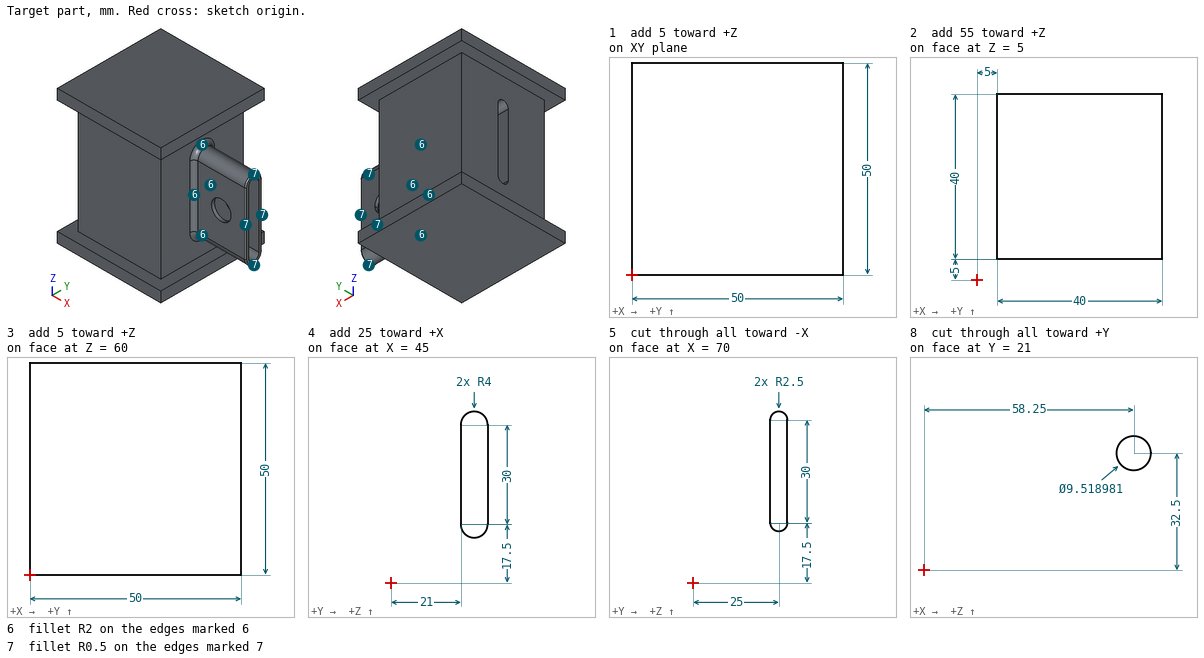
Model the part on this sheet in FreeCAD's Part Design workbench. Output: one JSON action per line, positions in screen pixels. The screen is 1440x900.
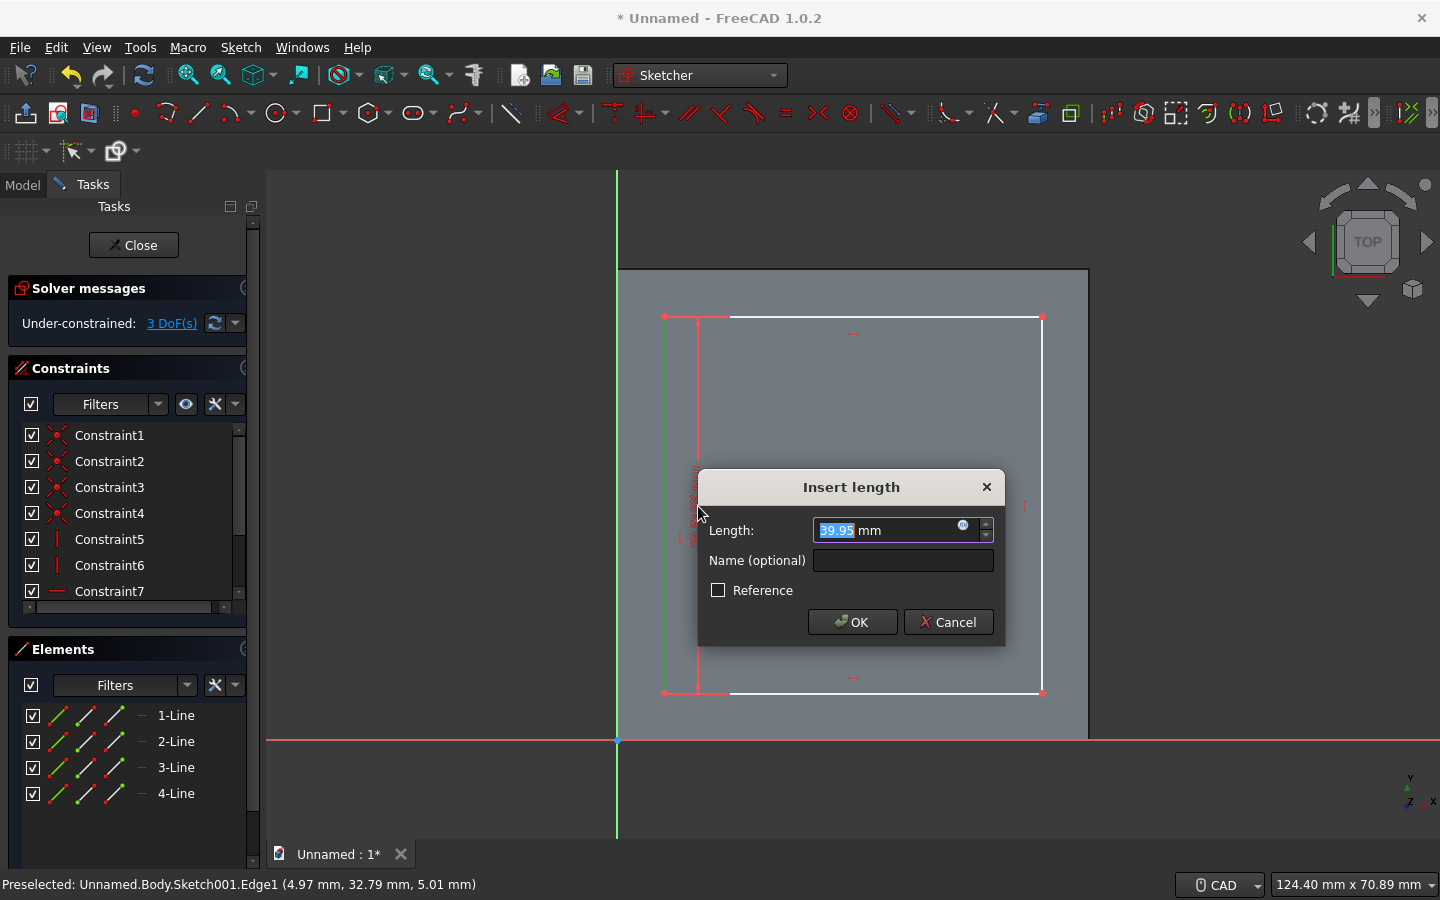
{"action": "type", "text": "40"}
{"action": "key", "text": "Return"}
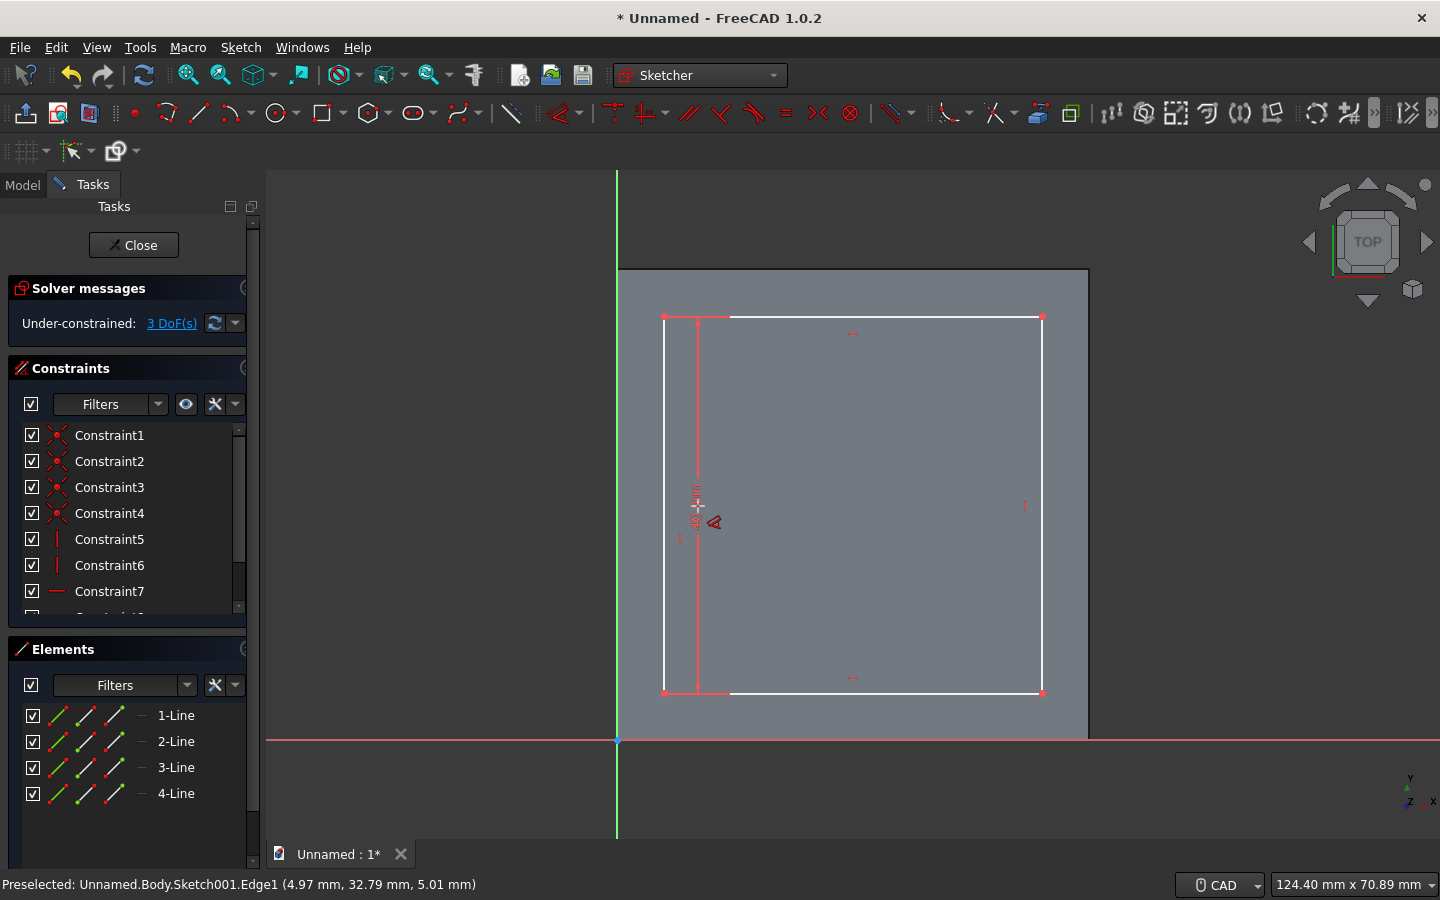
{"action": "left_click", "coordinate": [777, 694]}
{"action": "left_click", "coordinate": [853, 660]}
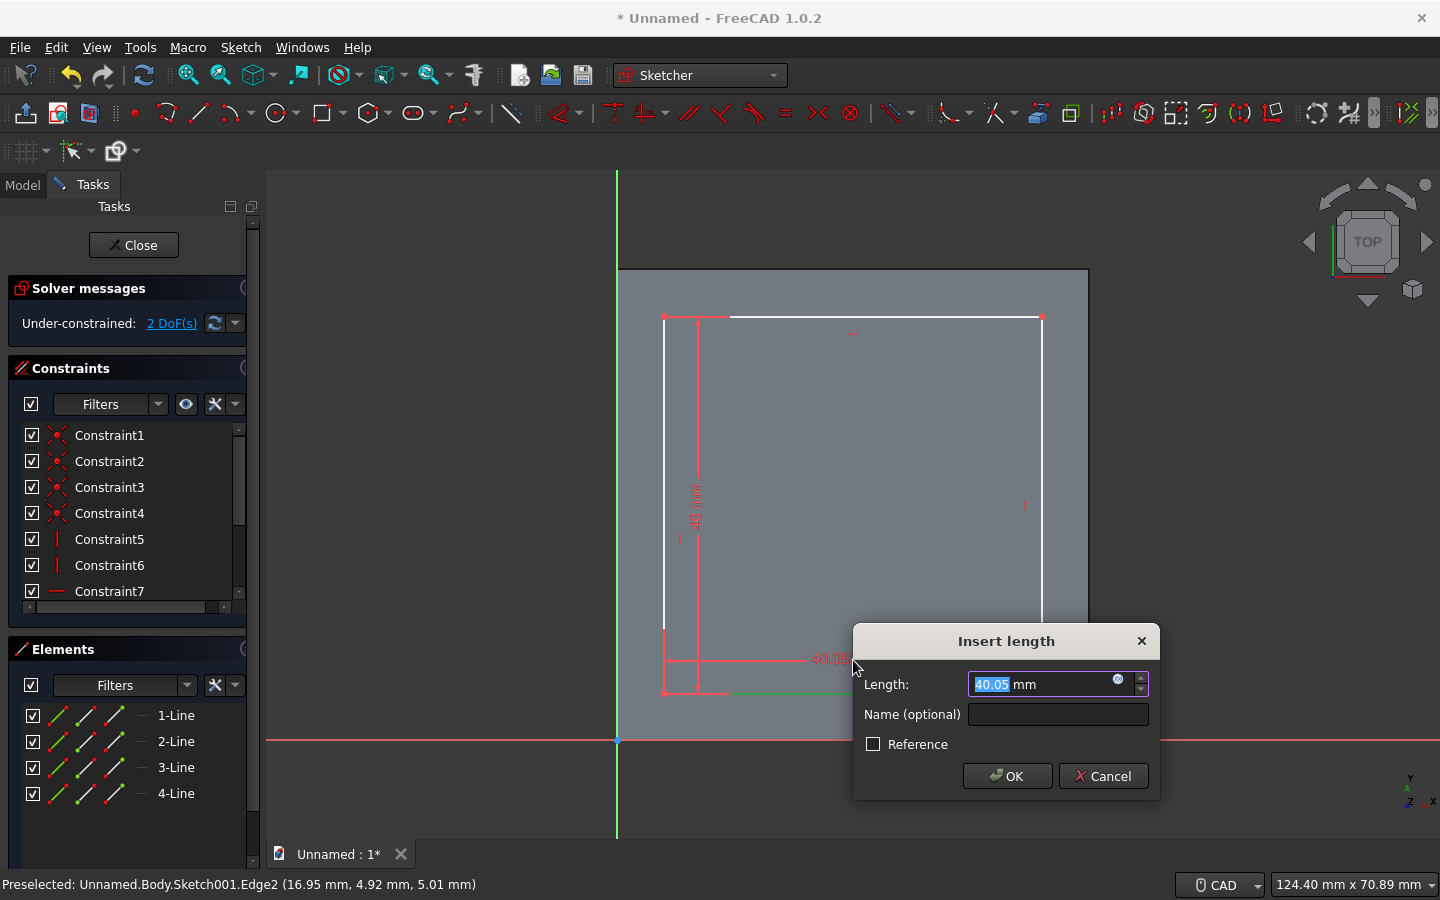
{"action": "type", "text": "40"}
{"action": "key", "text": "Return"}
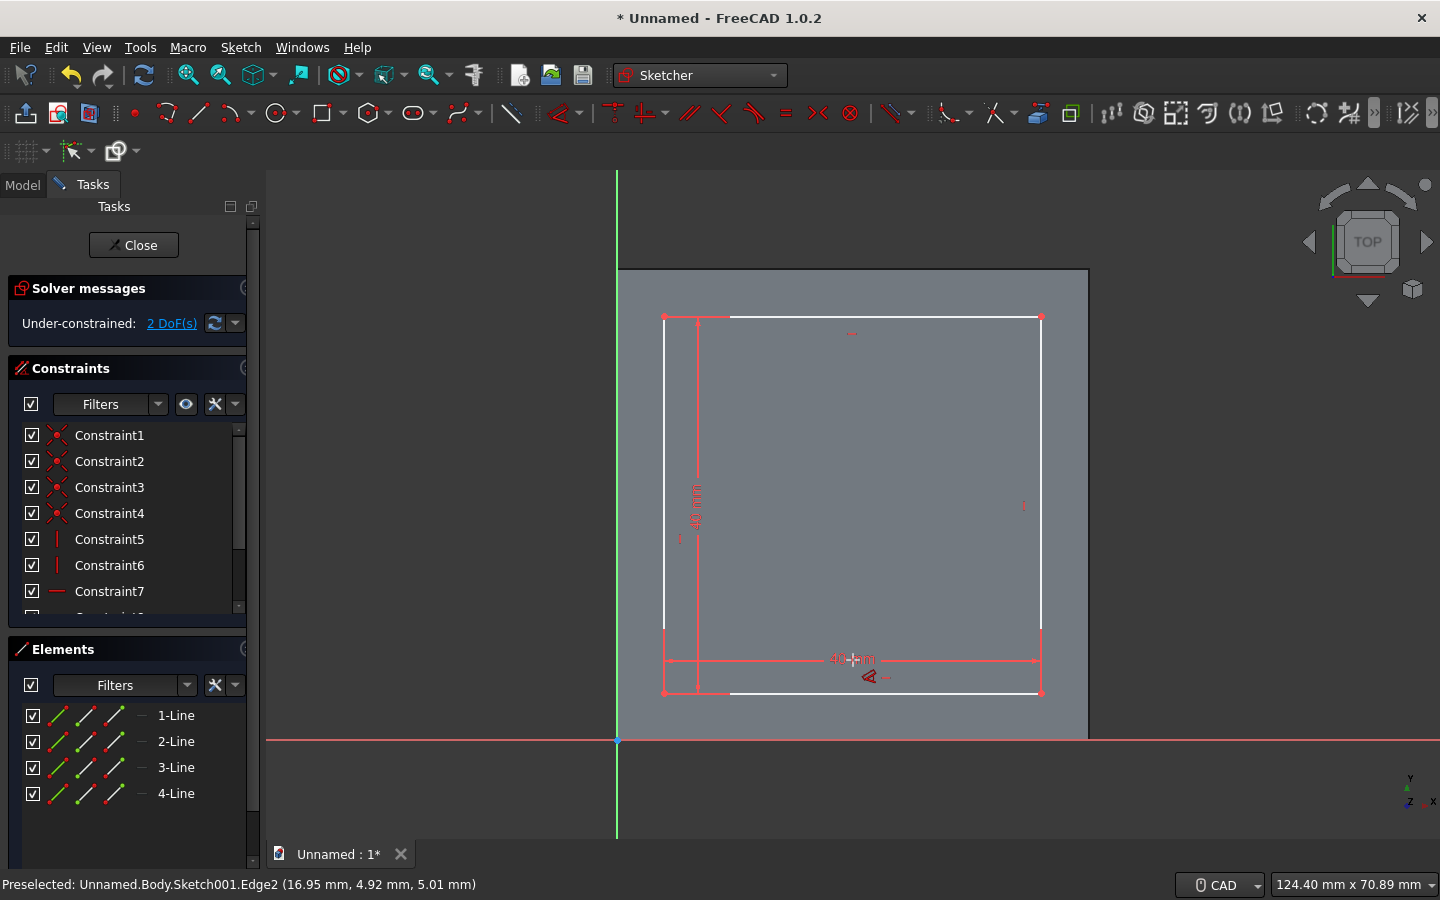
{"action": "left_click", "coordinate": [664, 316]}
{"action": "left_click", "coordinate": [641, 774]}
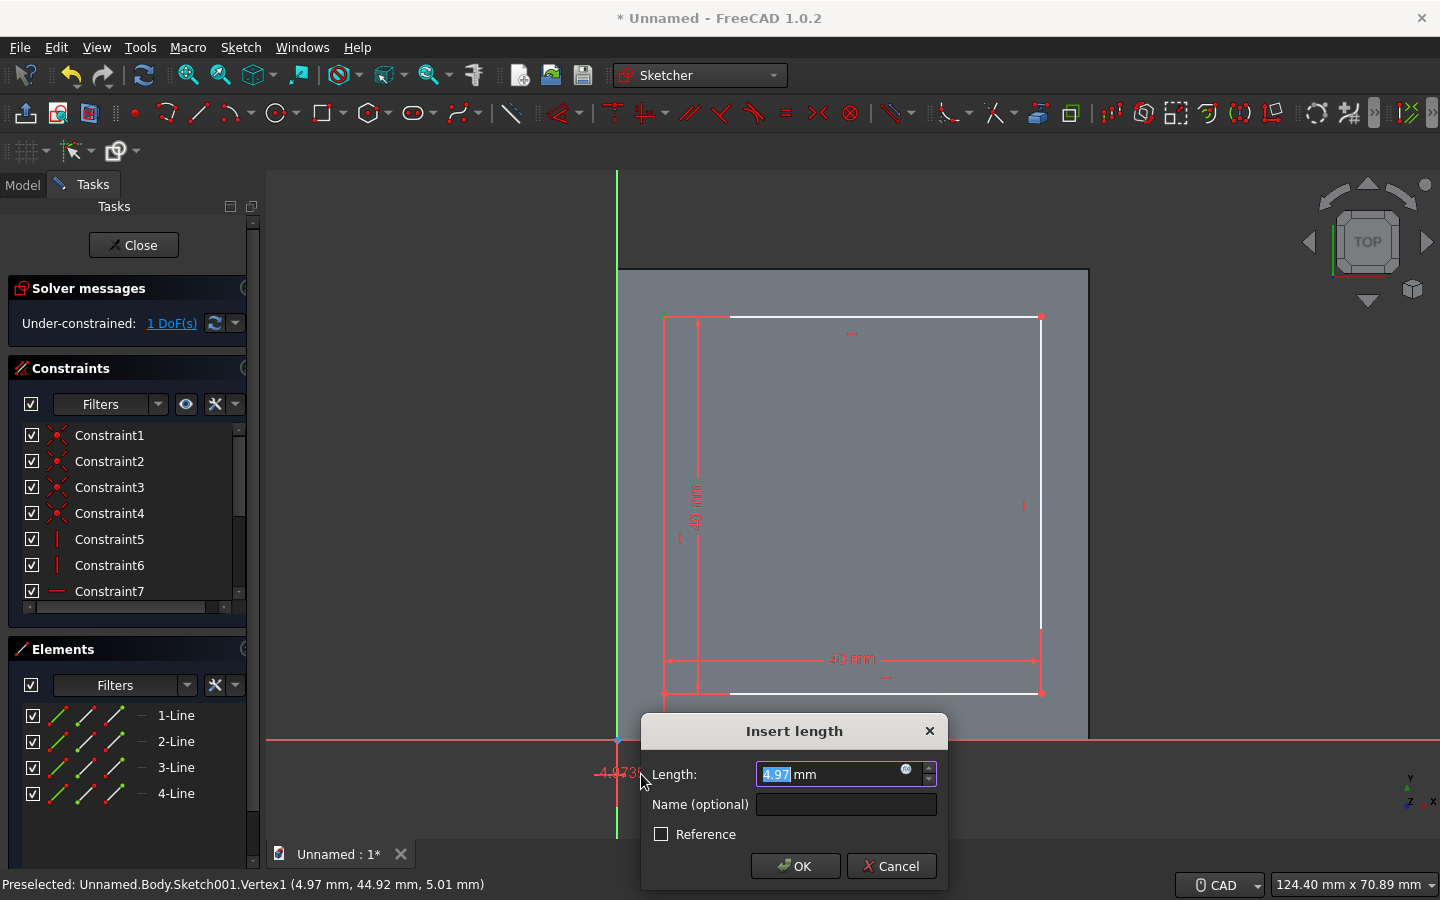
{"action": "type", "text": "5"}
{"action": "key", "text": "Return"}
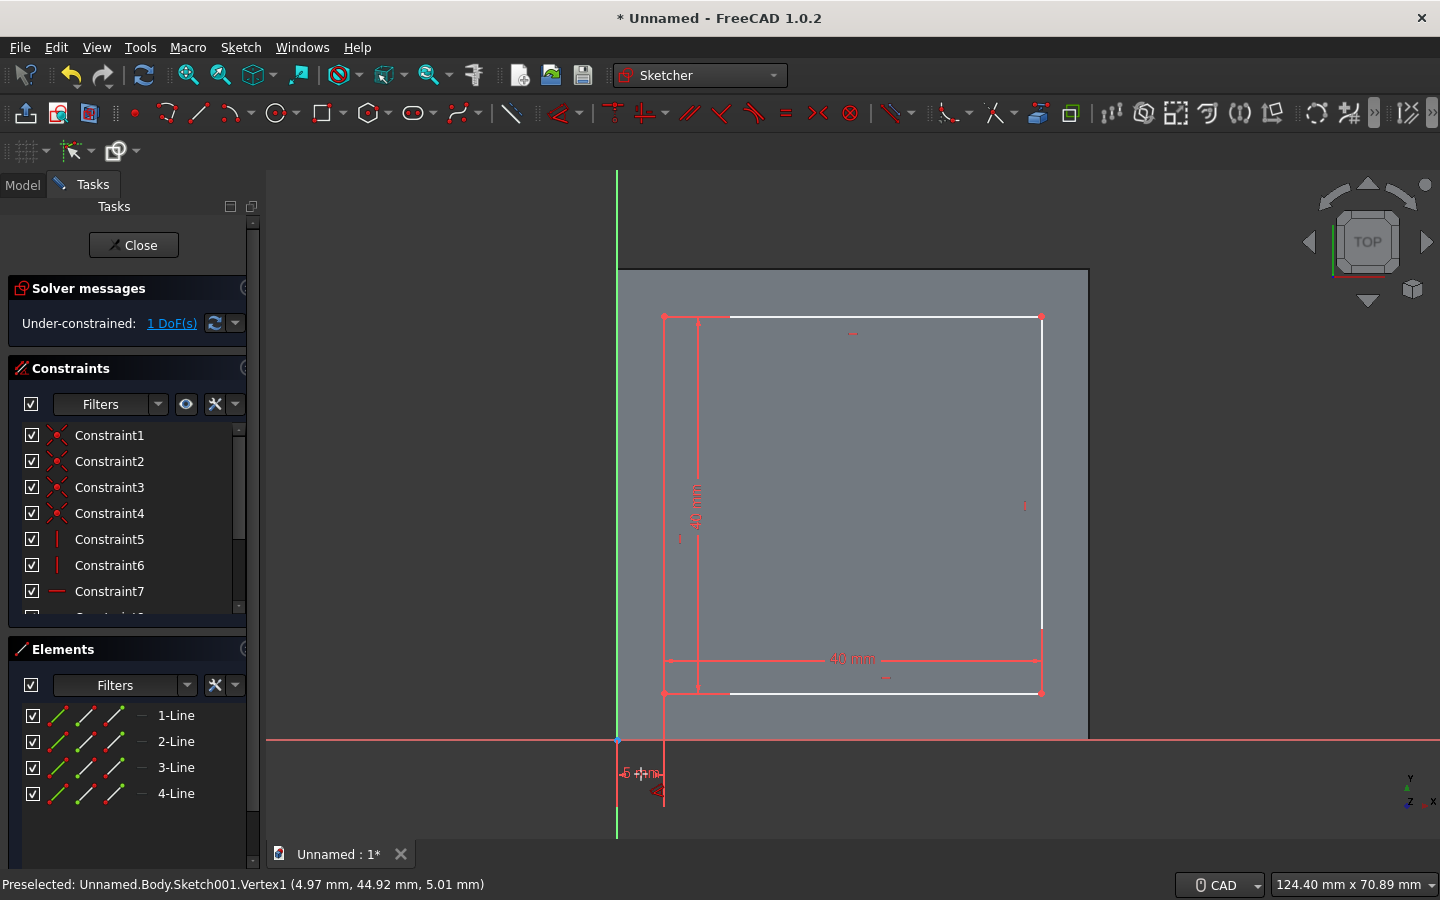
{"action": "left_click", "coordinate": [664, 694]}
{"action": "left_click", "coordinate": [583, 717]}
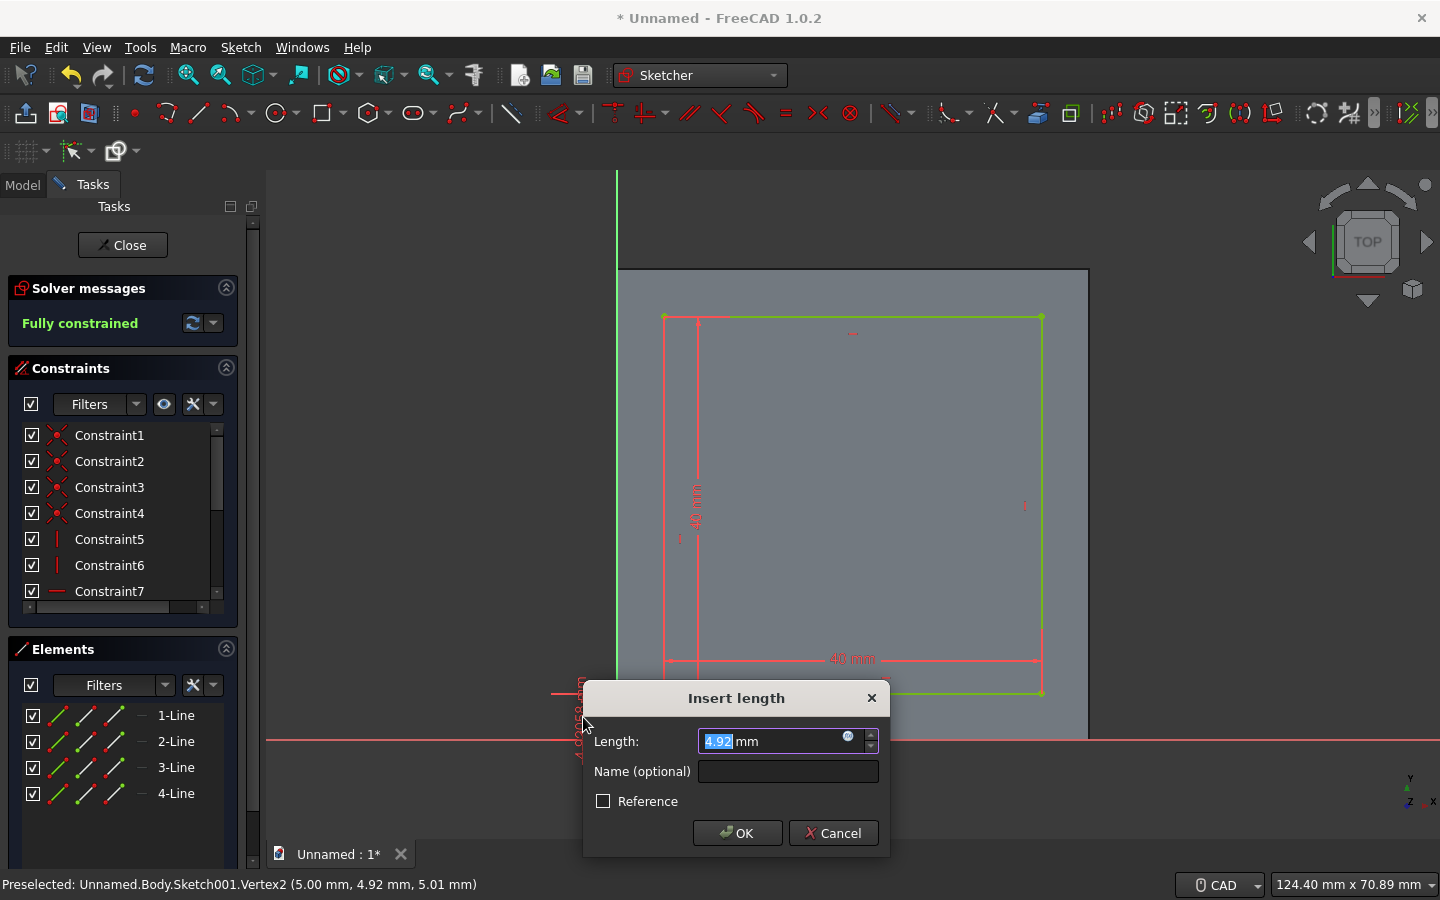
{"action": "type", "text": "5"}
{"action": "key", "text": "Return"}
{"action": "key", "text": "Escape"}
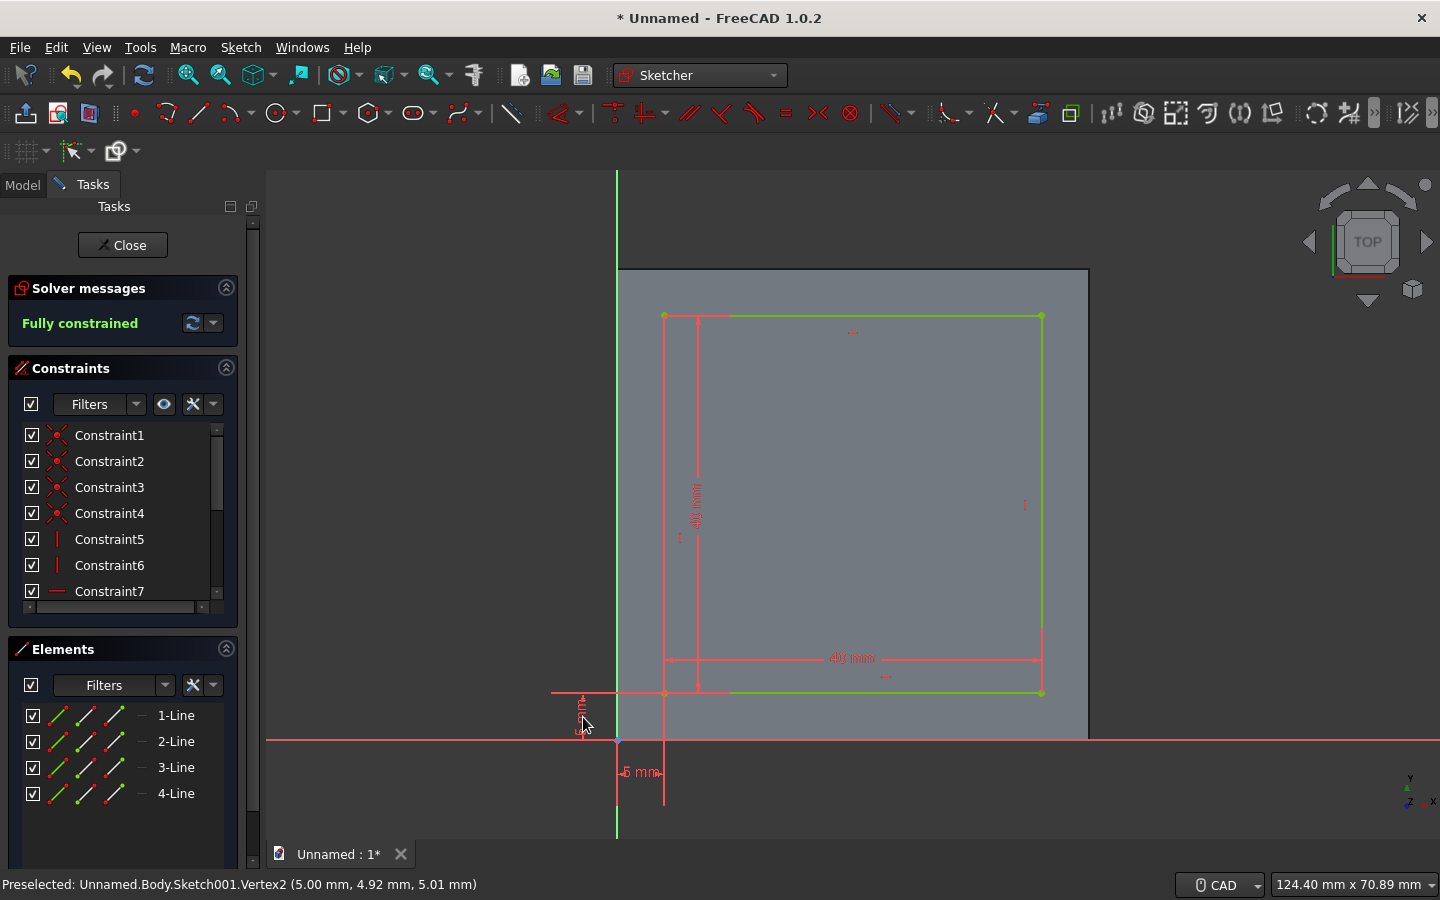
{"action": "left_click", "coordinate": [123, 245]}